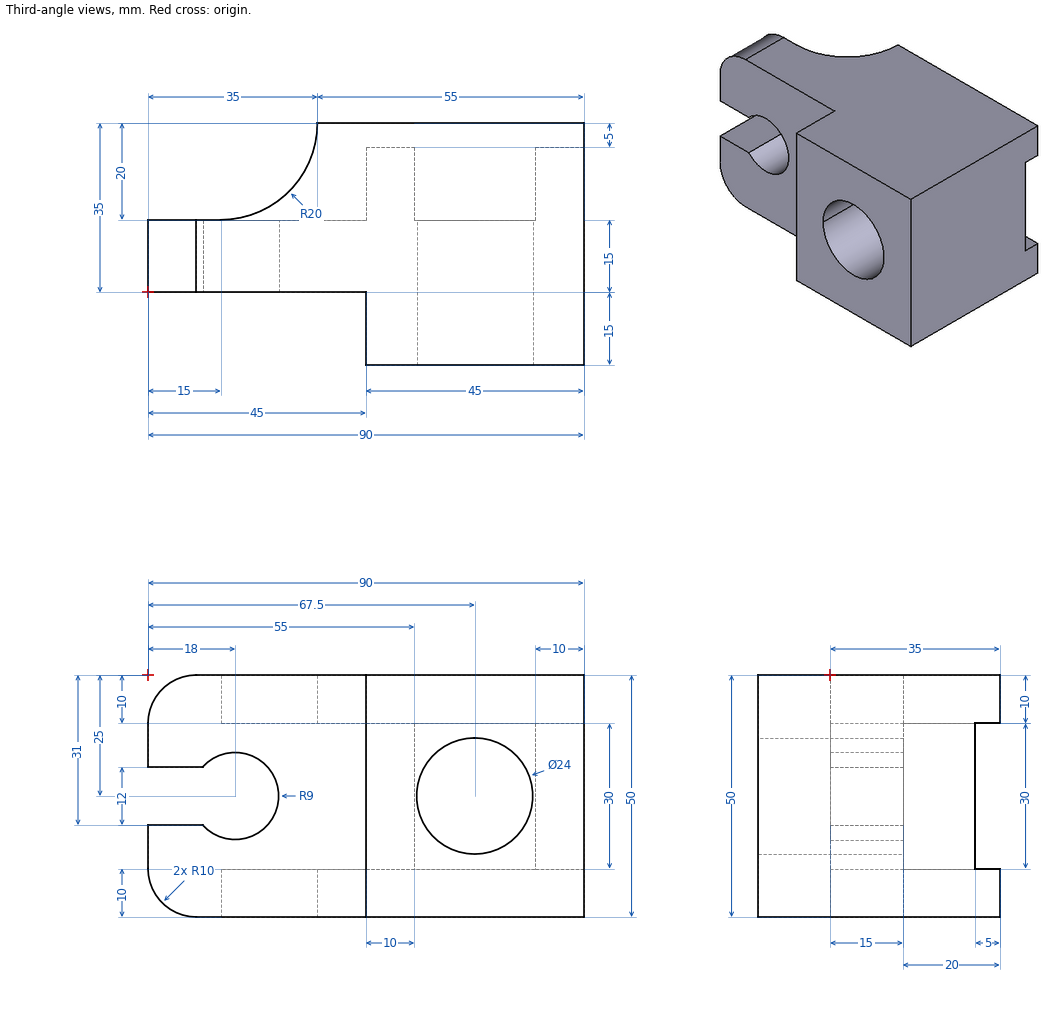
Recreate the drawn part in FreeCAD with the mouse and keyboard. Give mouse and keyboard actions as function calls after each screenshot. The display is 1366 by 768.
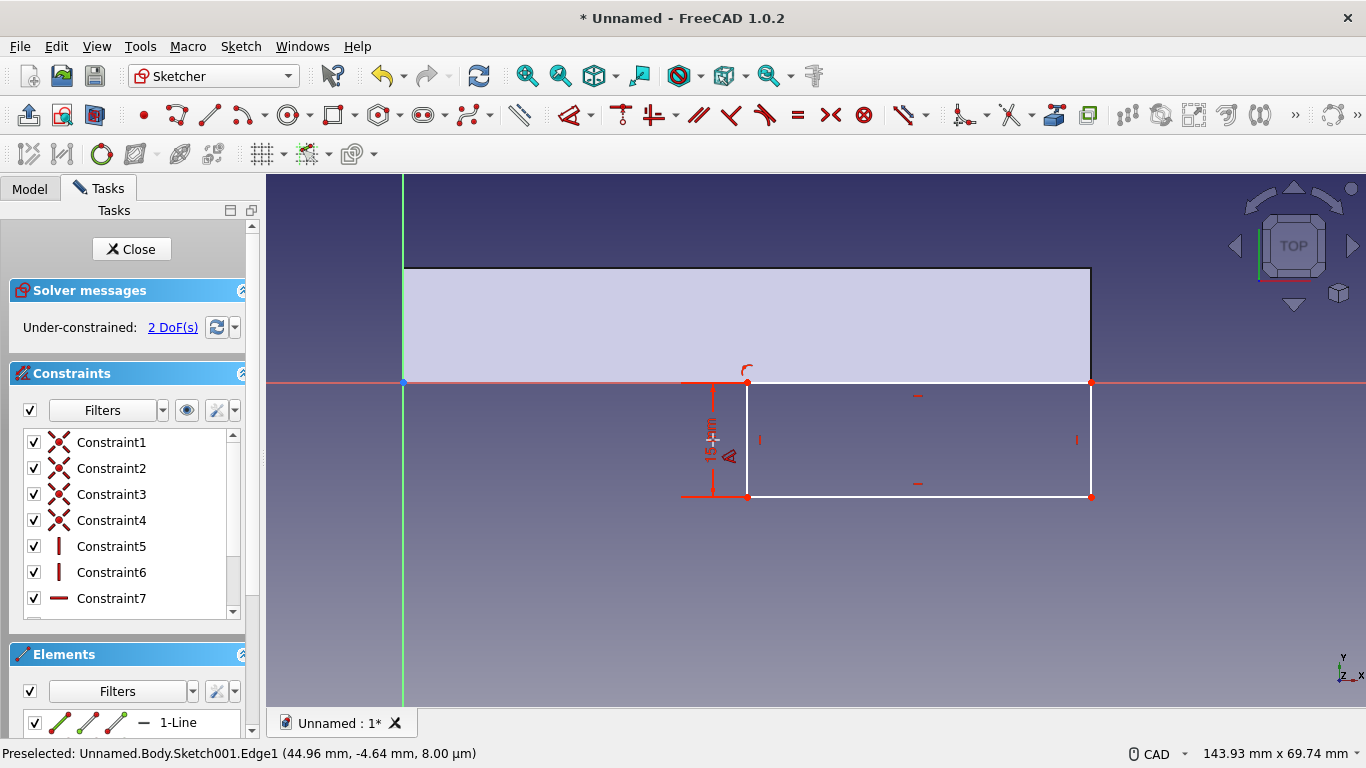
click(850, 497)
click(919, 531)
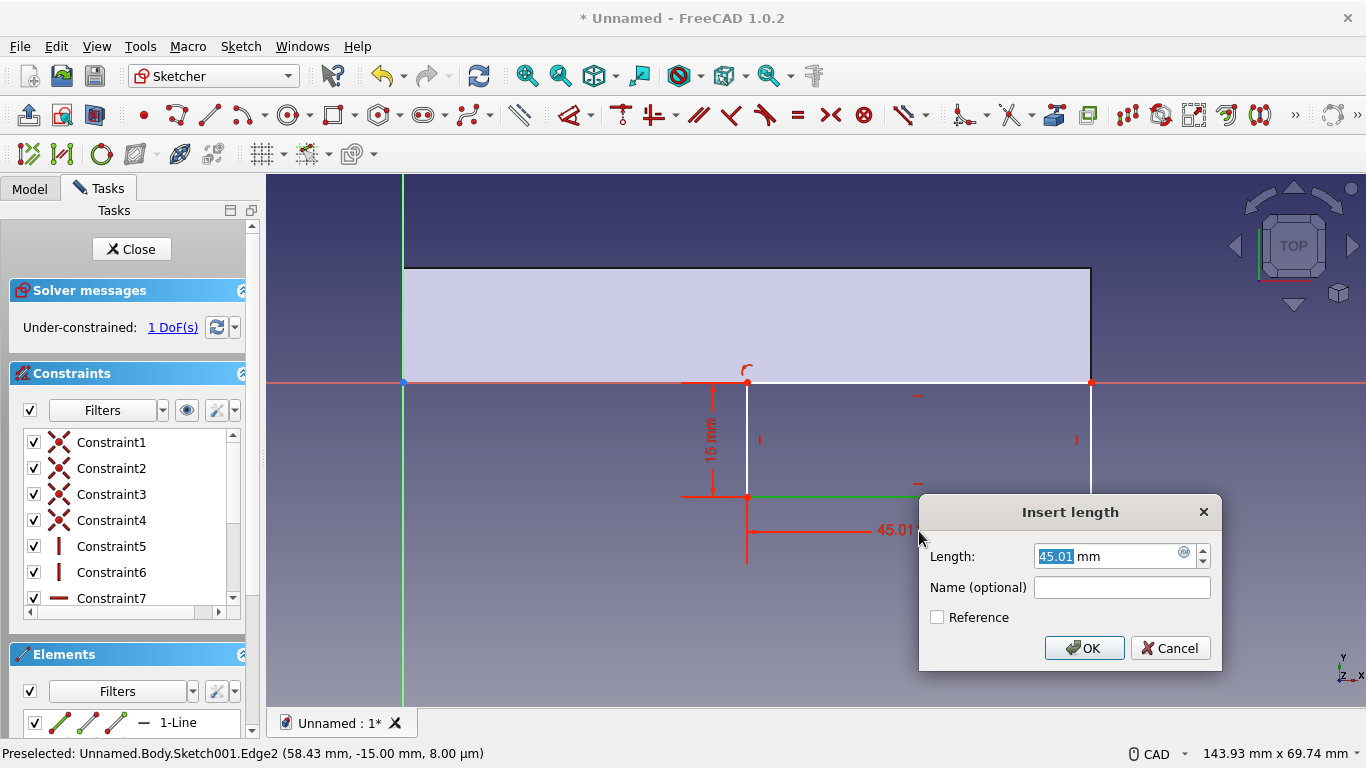
text(45)
key(Return)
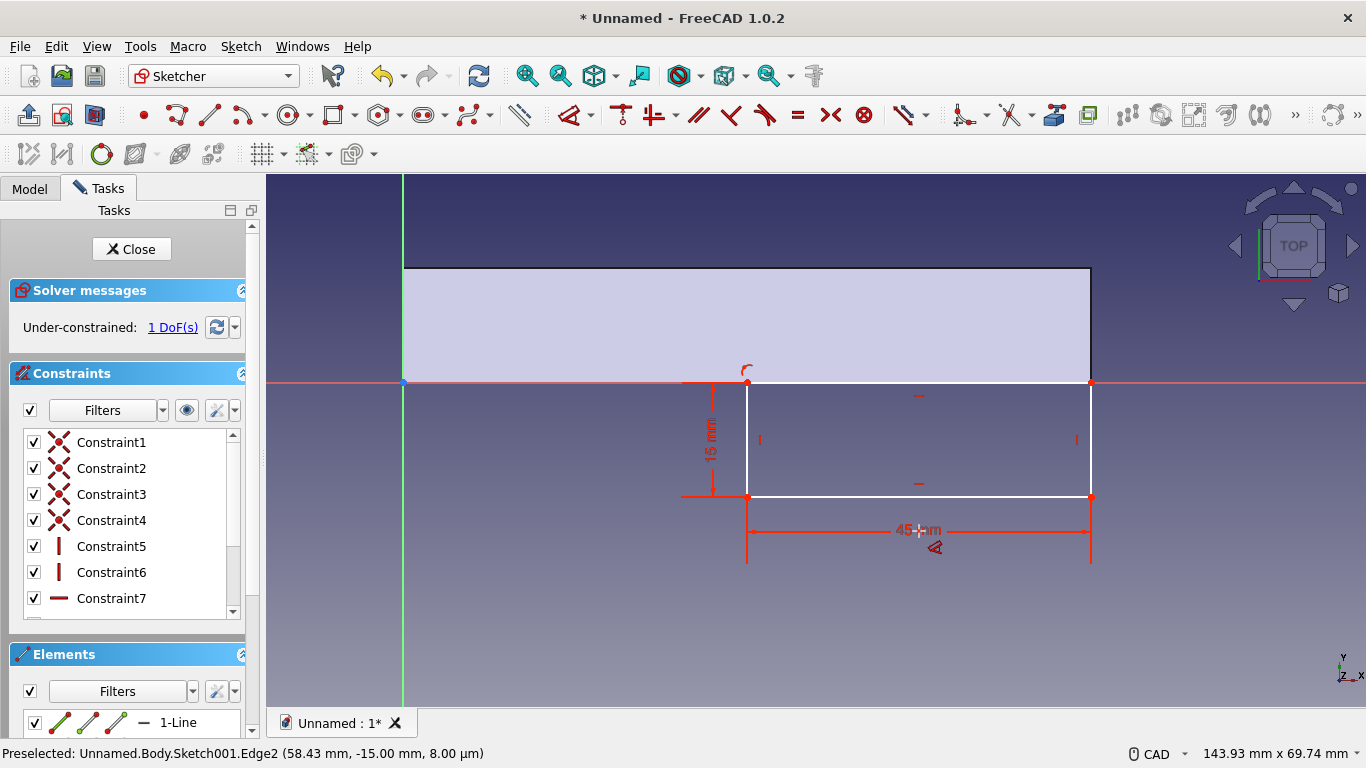
click(747, 383)
click(575, 349)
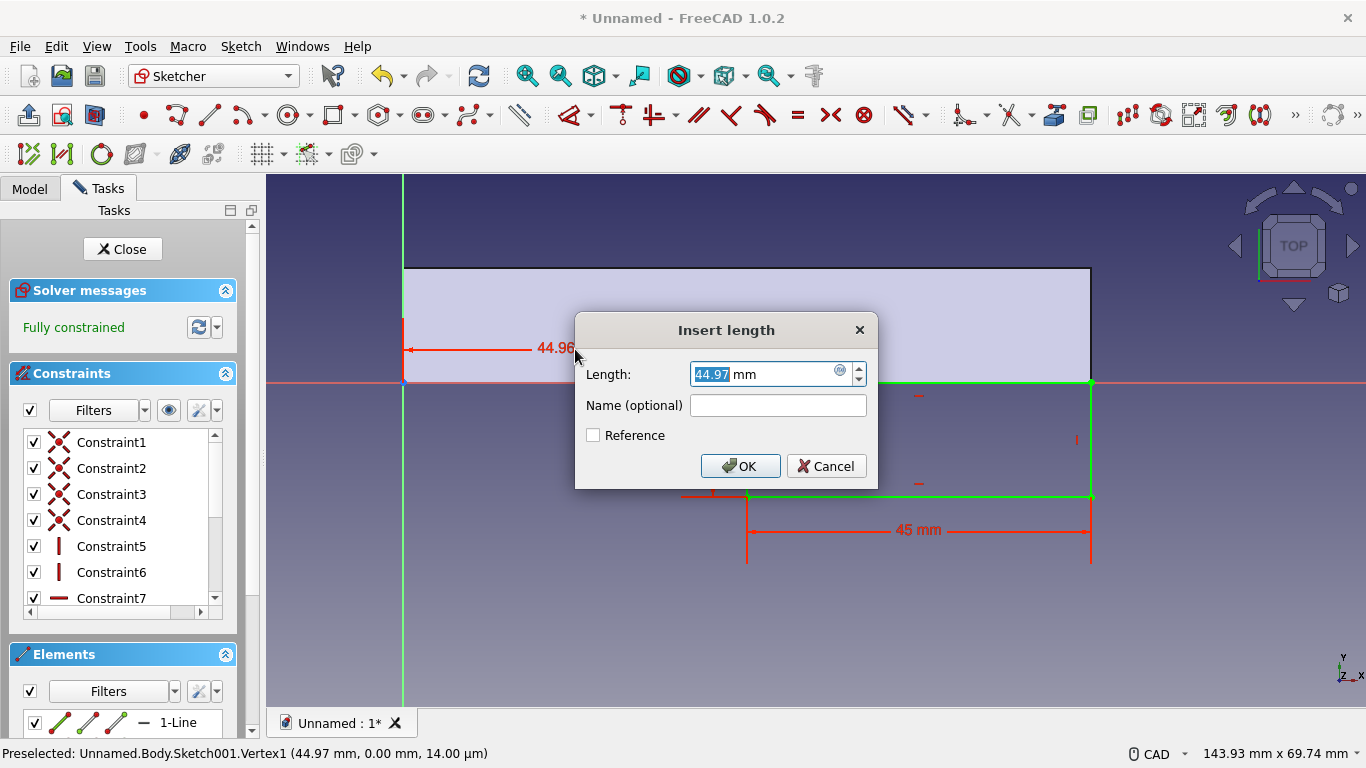
text(45)
key(Return)
key(Escape)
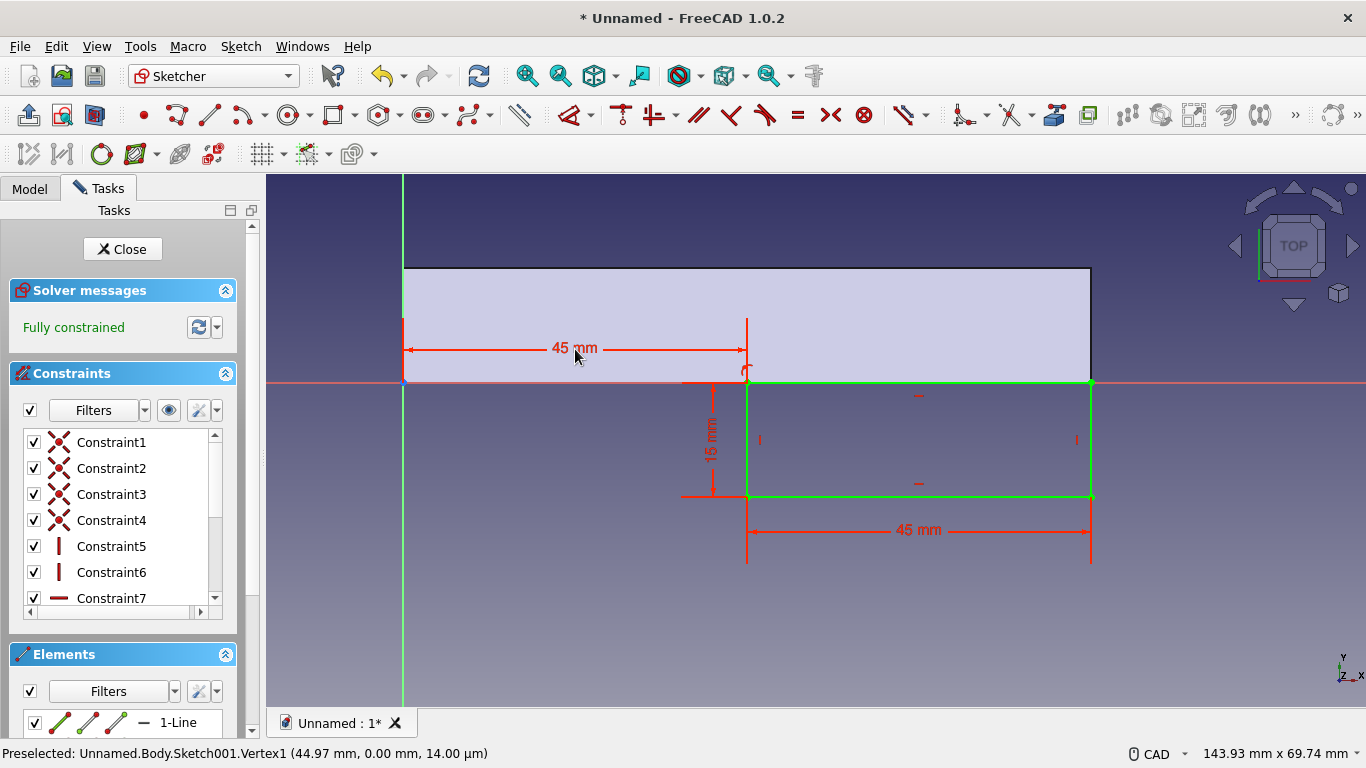
click(123, 249)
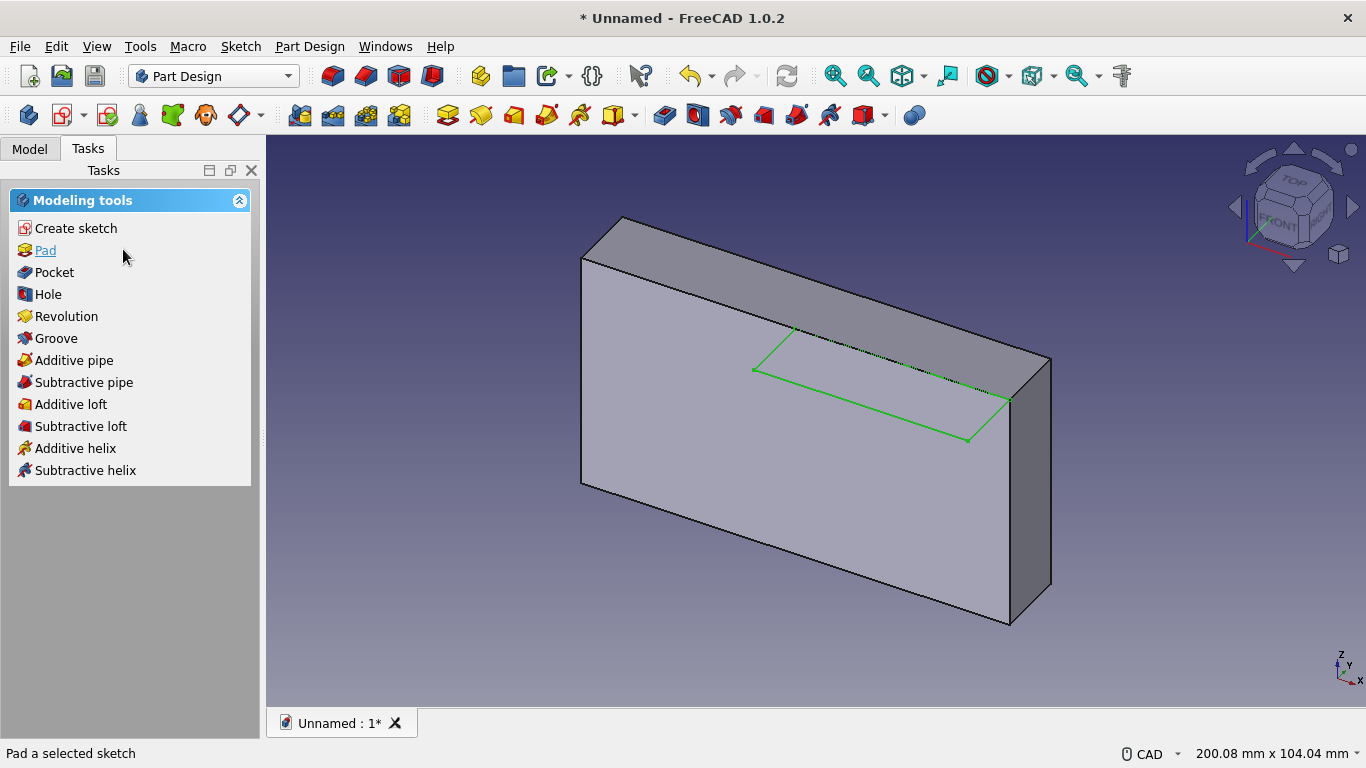
click(448, 116)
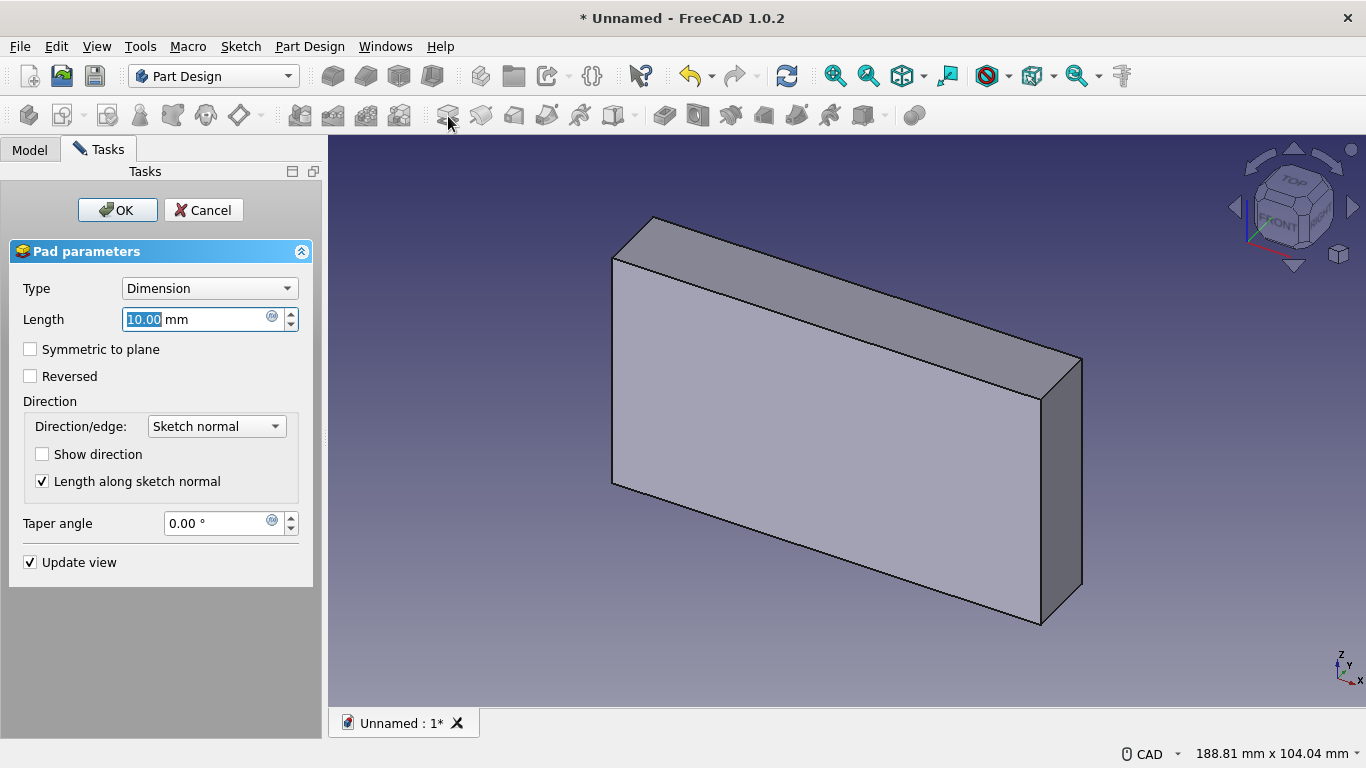
text(50)
key(Tab)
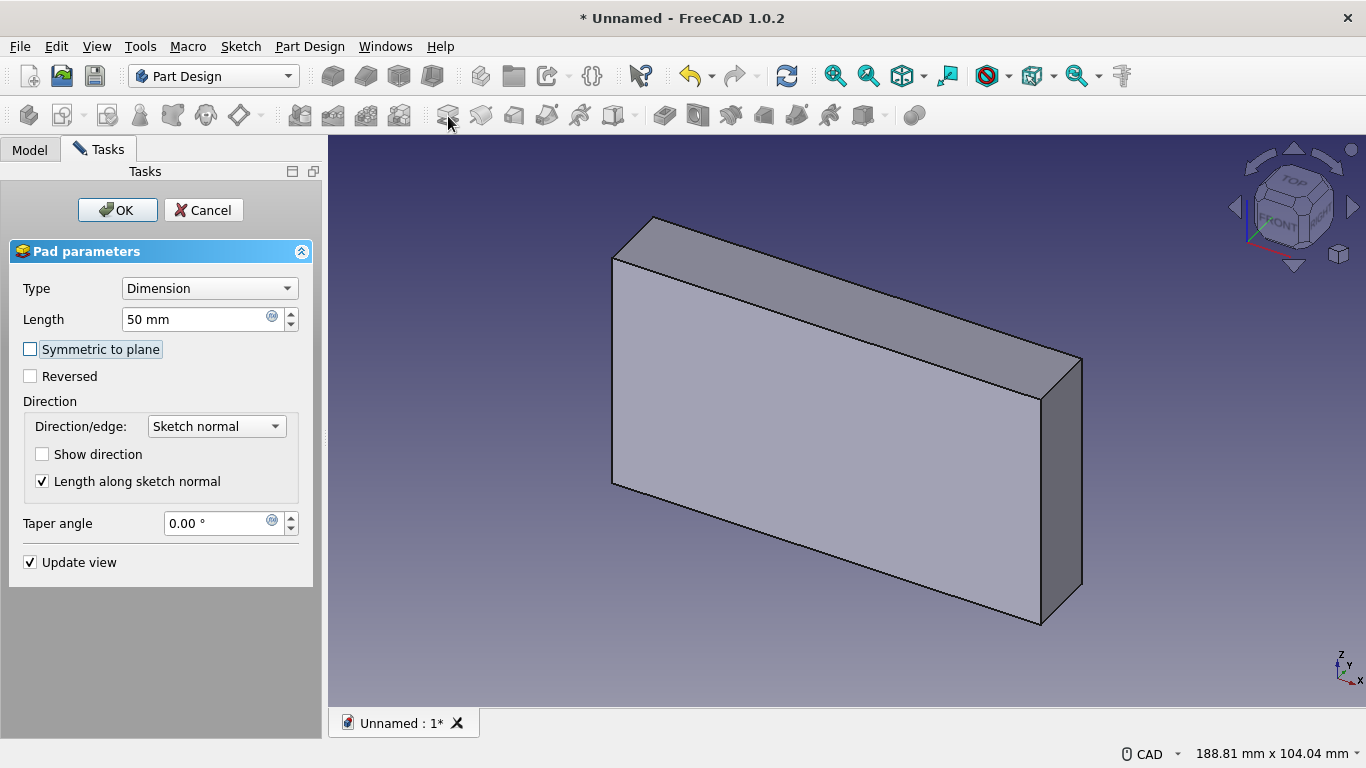
click(31, 376)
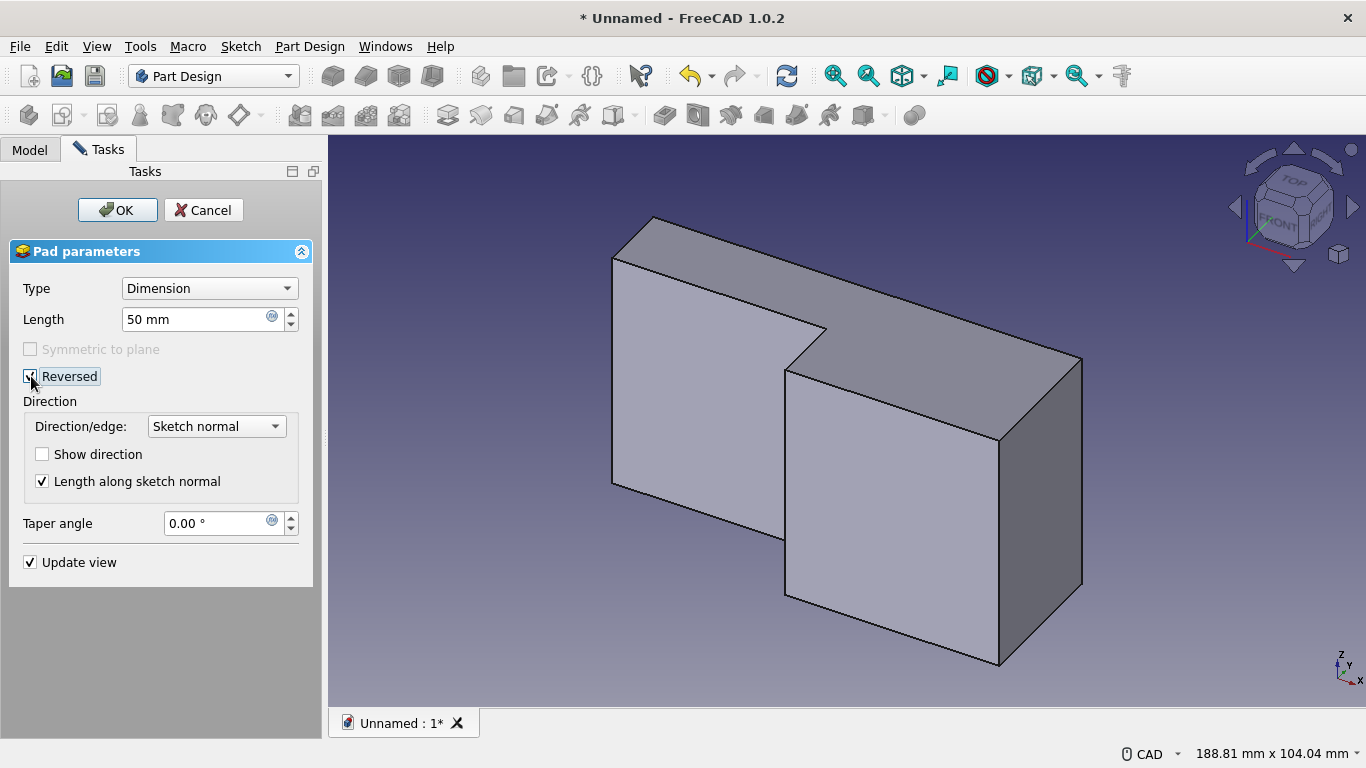
click(118, 210)